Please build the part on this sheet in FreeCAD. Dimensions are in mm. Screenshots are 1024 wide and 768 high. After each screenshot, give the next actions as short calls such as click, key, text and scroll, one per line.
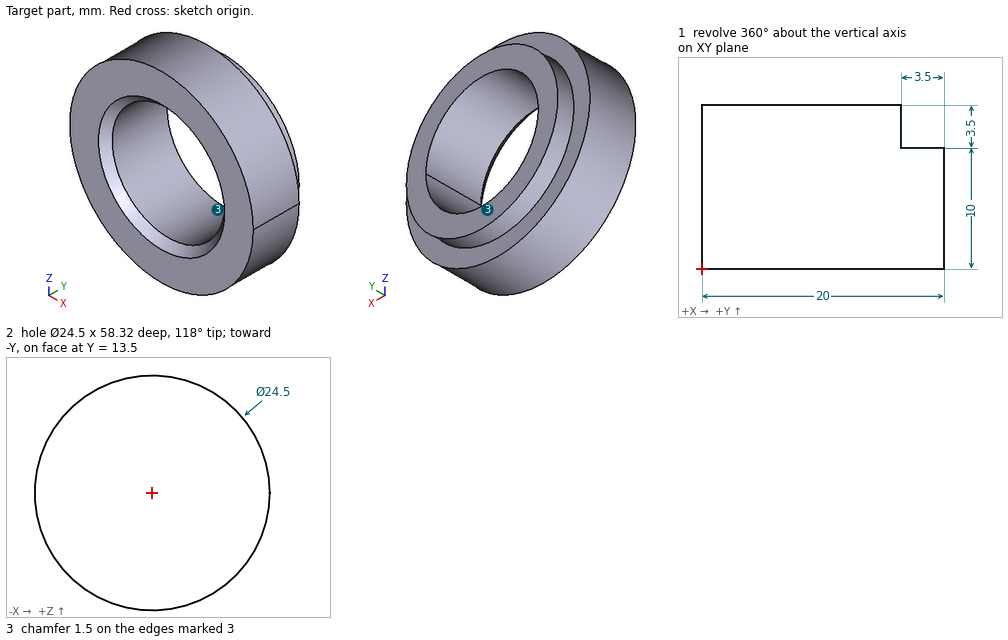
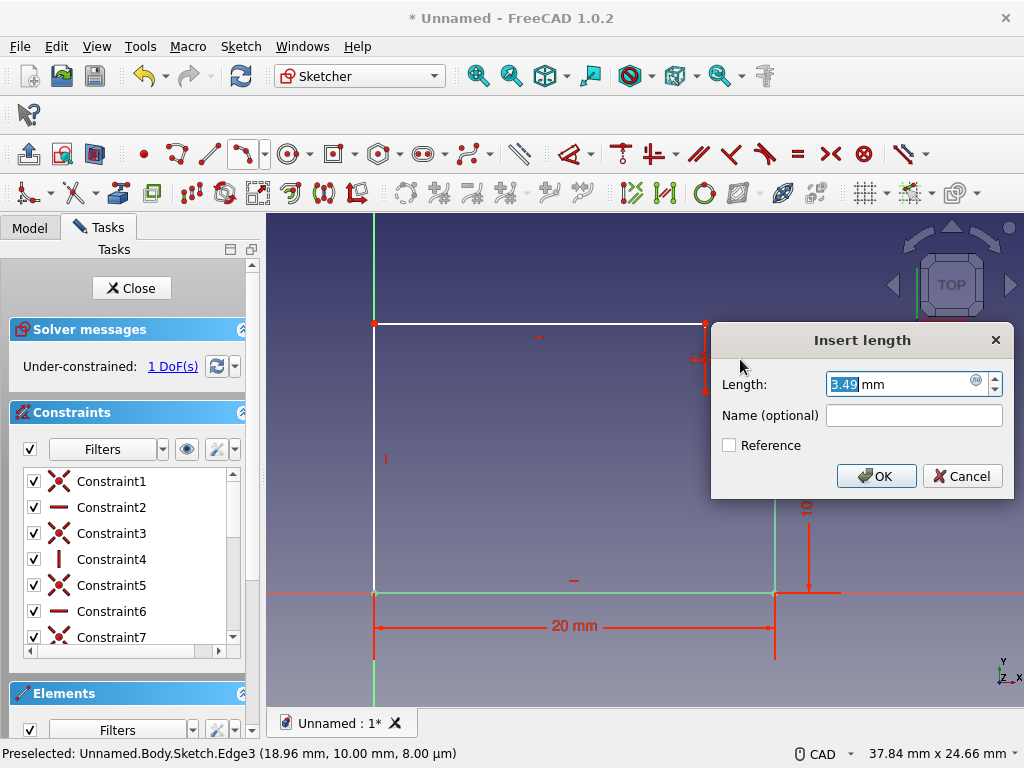
text(3.5)
key(Return)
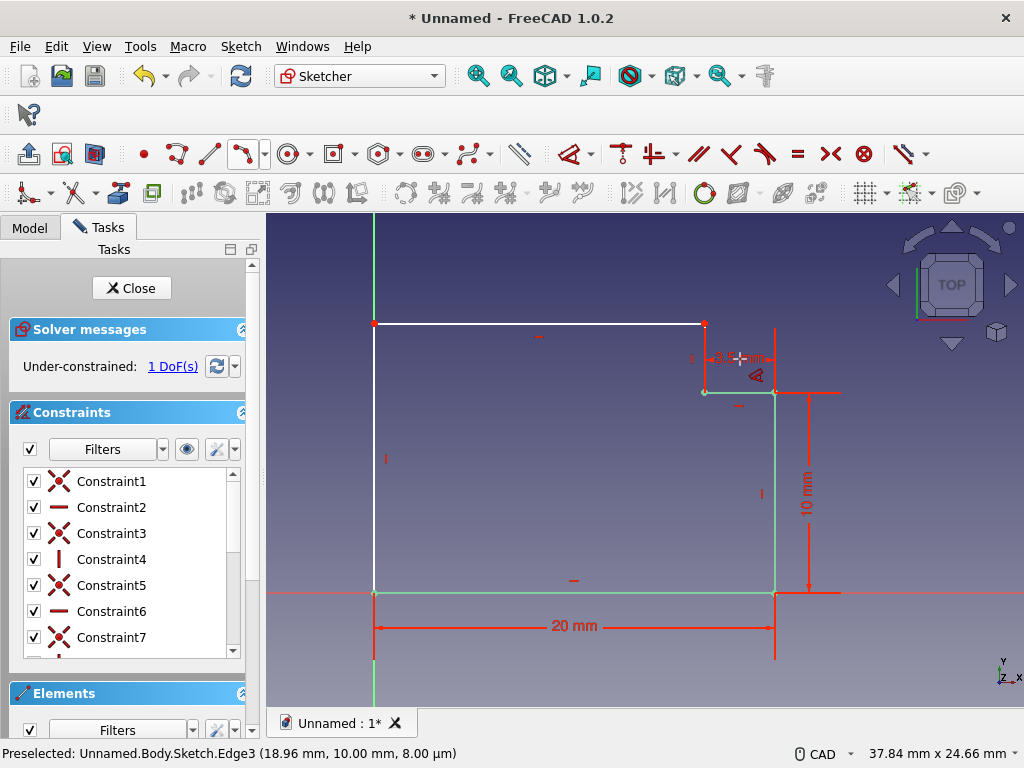
click(705, 372)
click(739, 334)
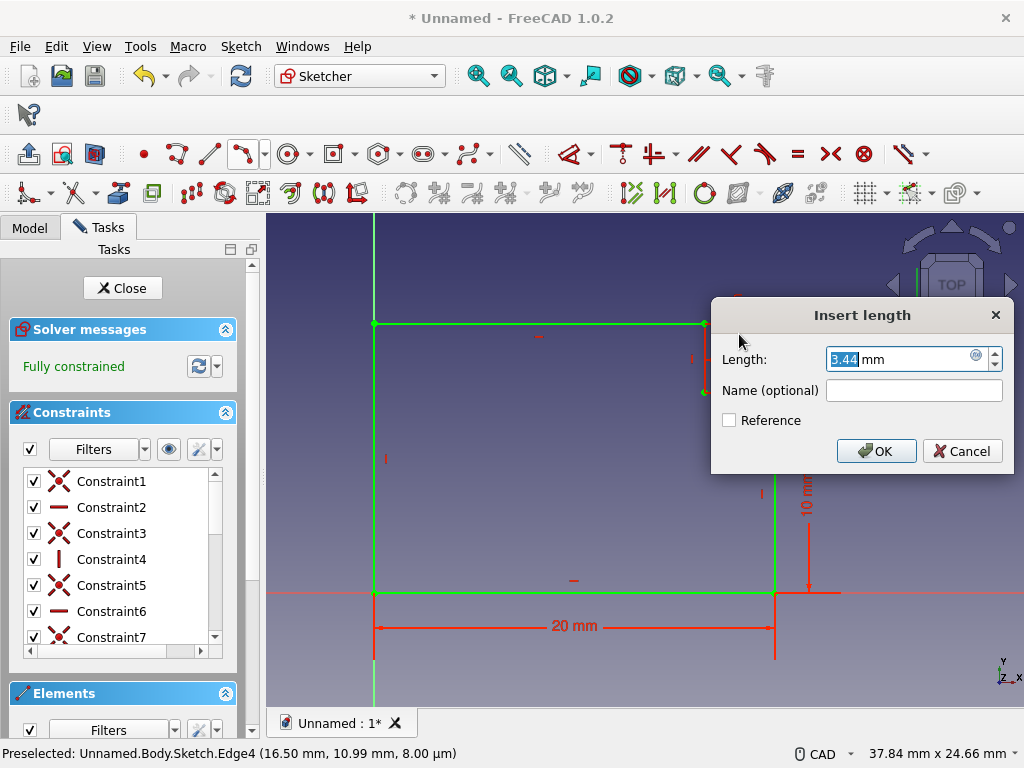
text(3.5)
key(Return)
key(Escape)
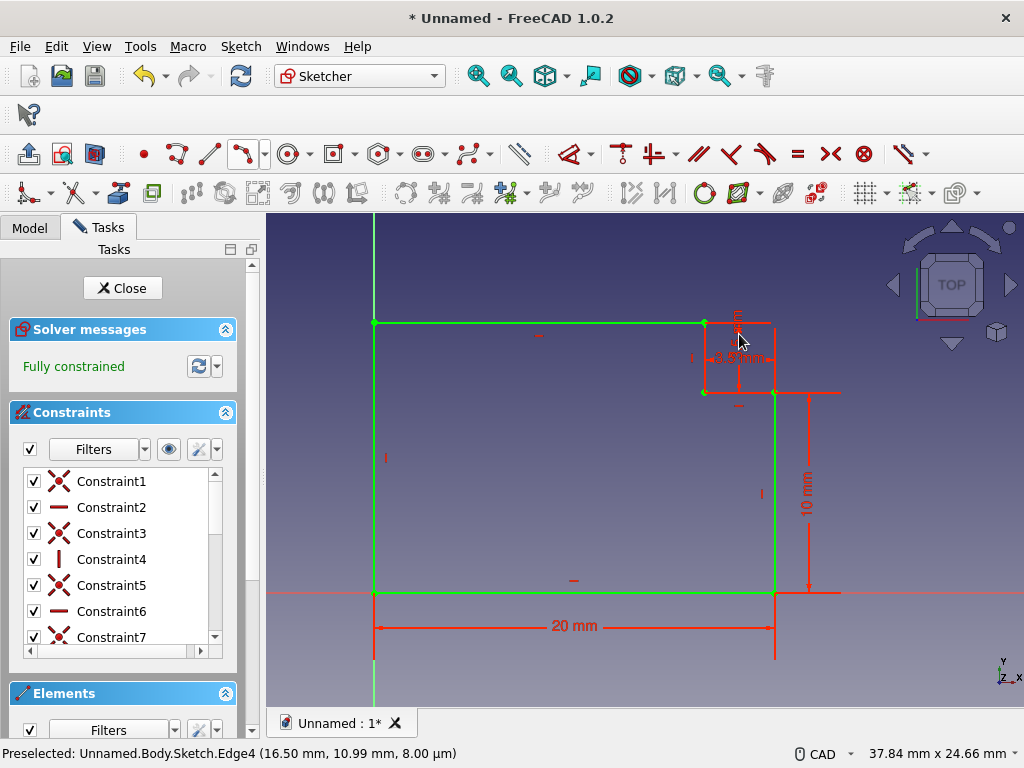
click(123, 288)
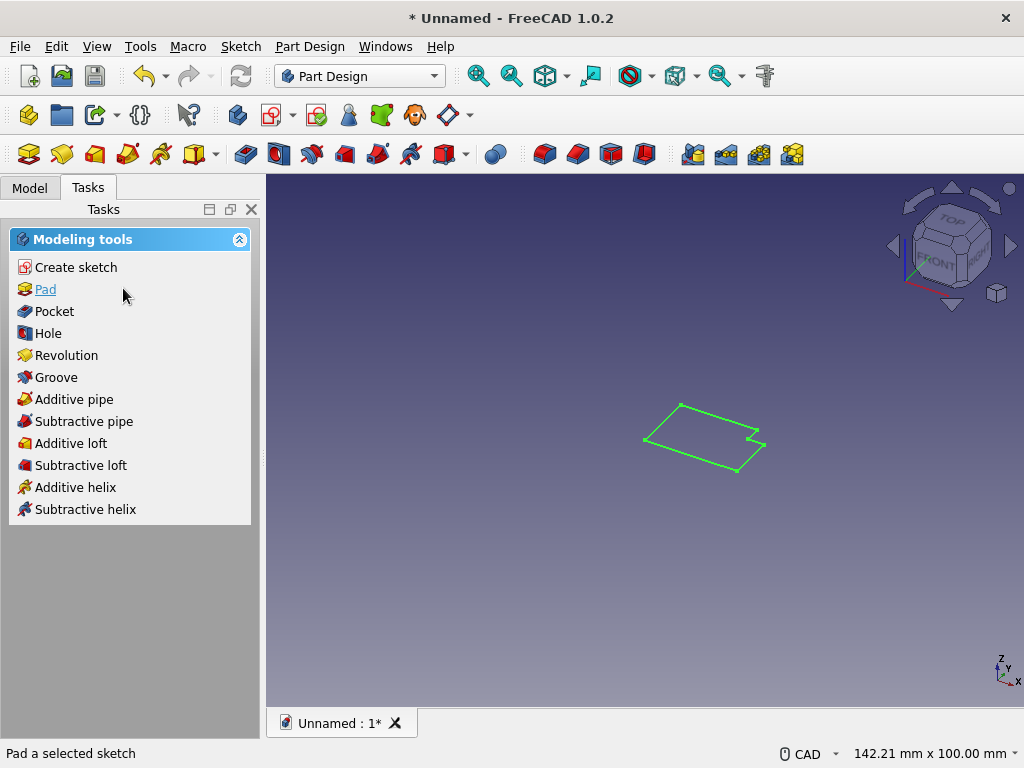
click(62, 154)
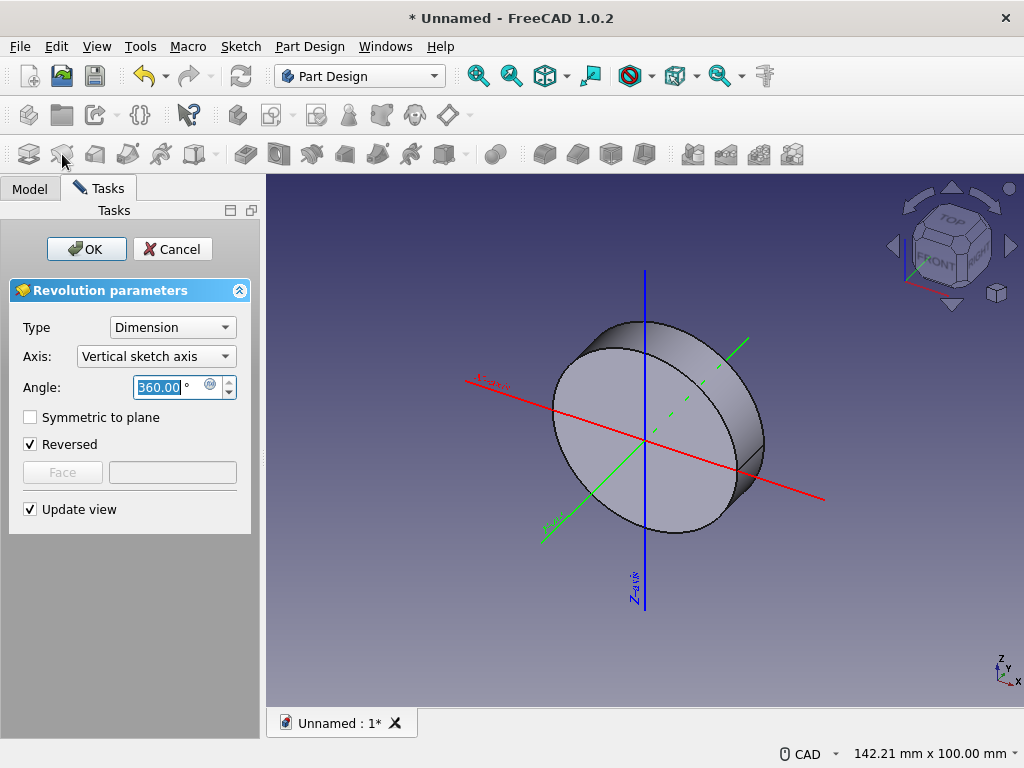
click(87, 249)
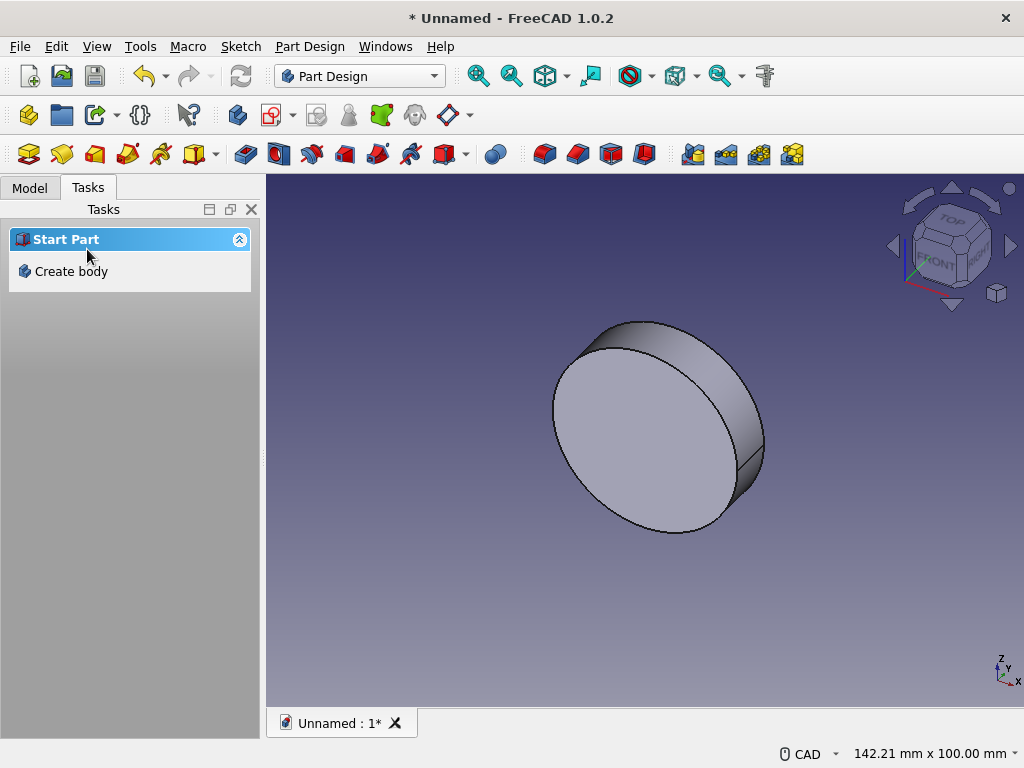
key(4)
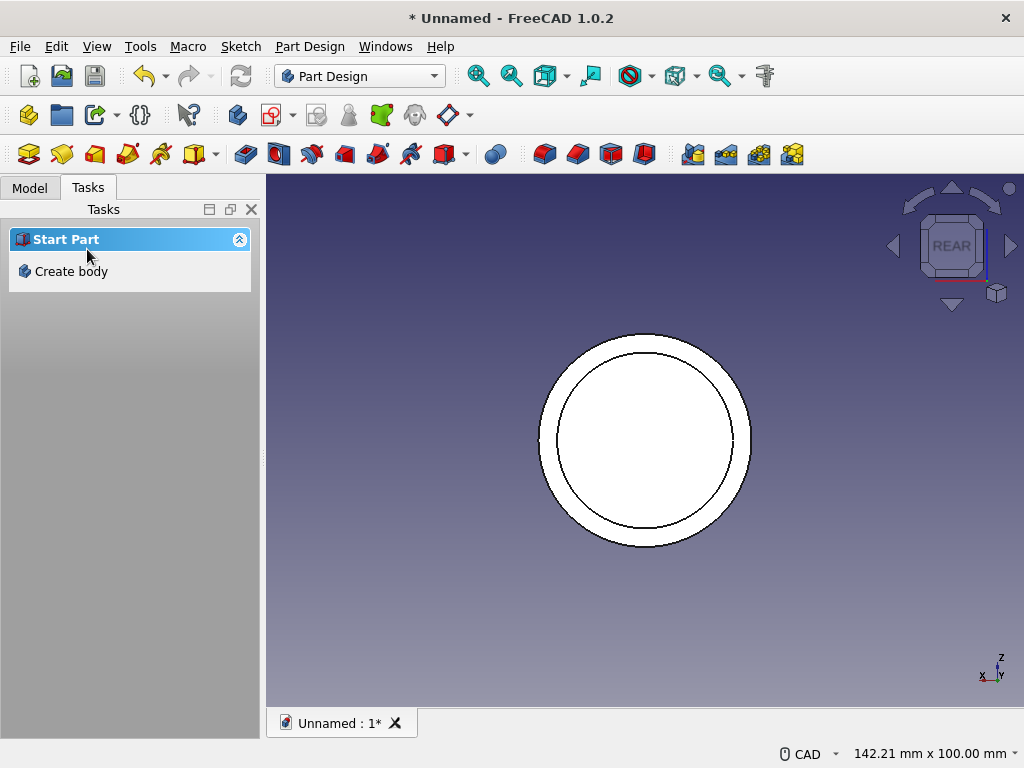
click(479, 76)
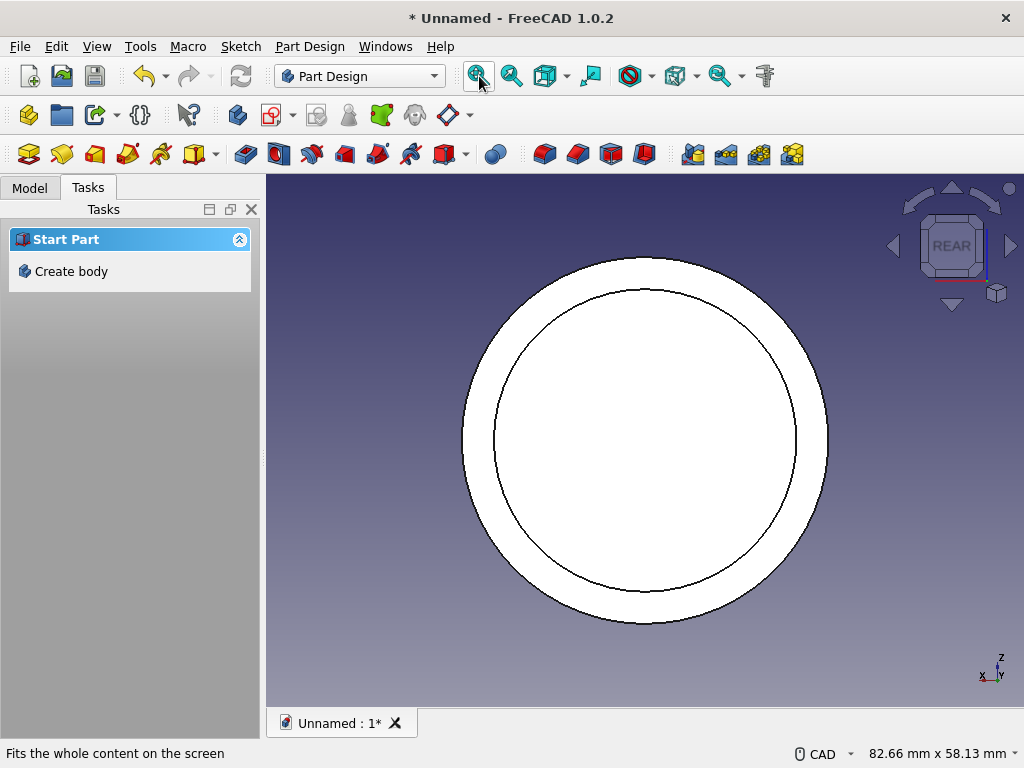
click(645, 440)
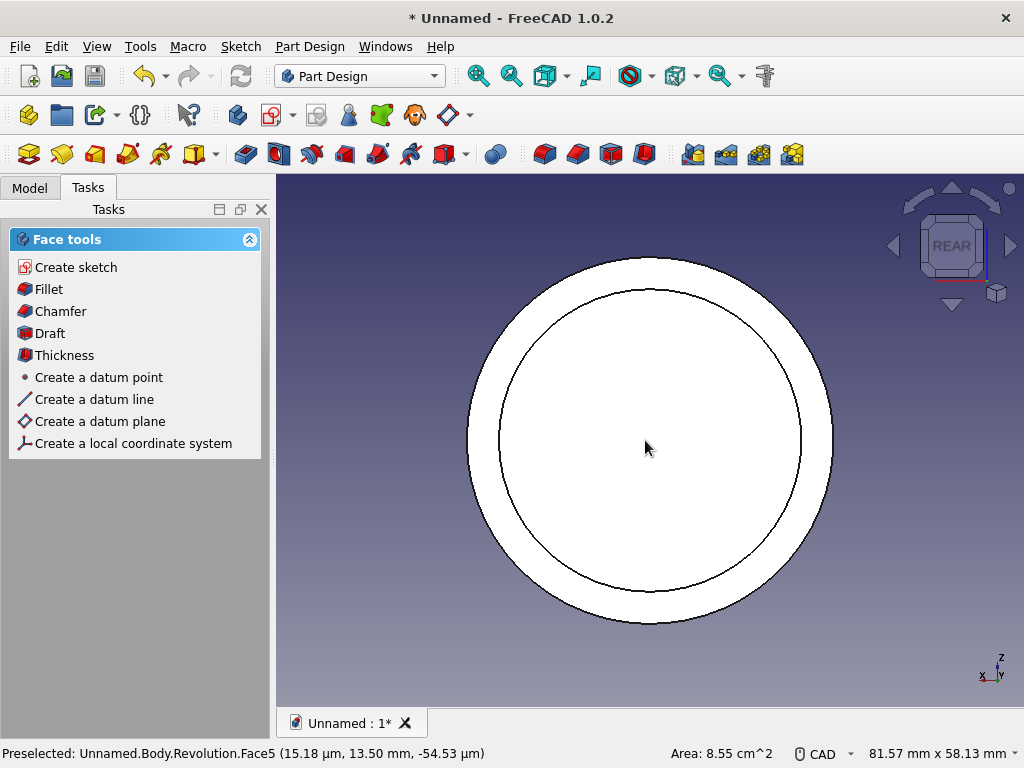
click(270, 116)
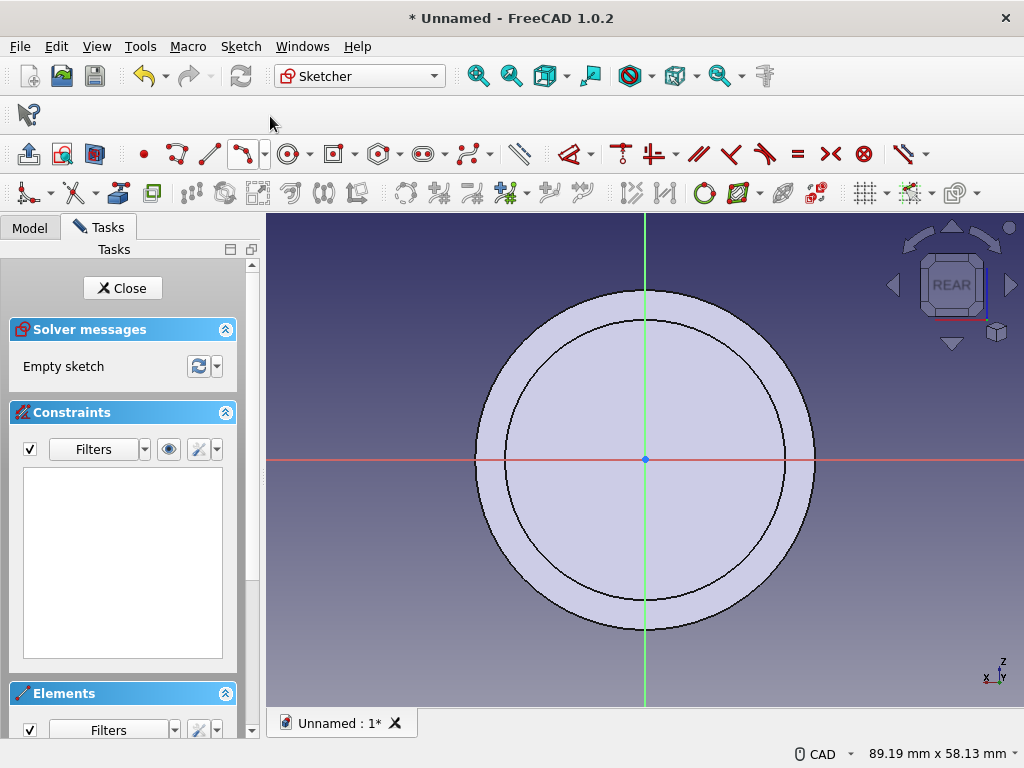
scroll(785, 460, up, 2)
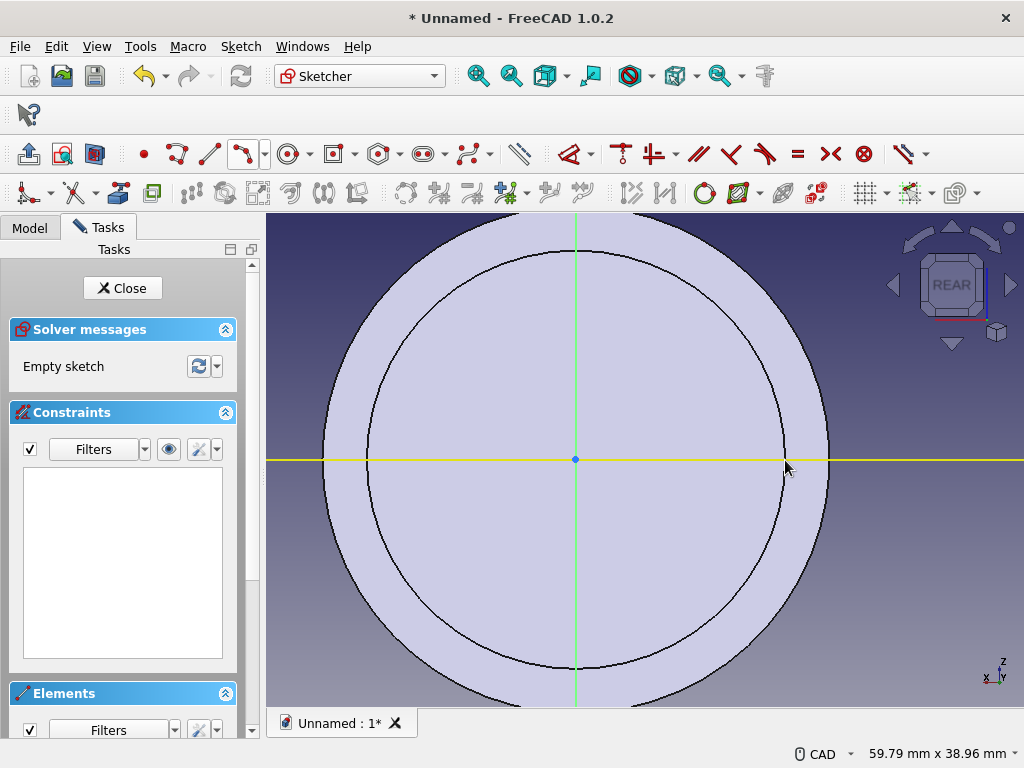
click(288, 154)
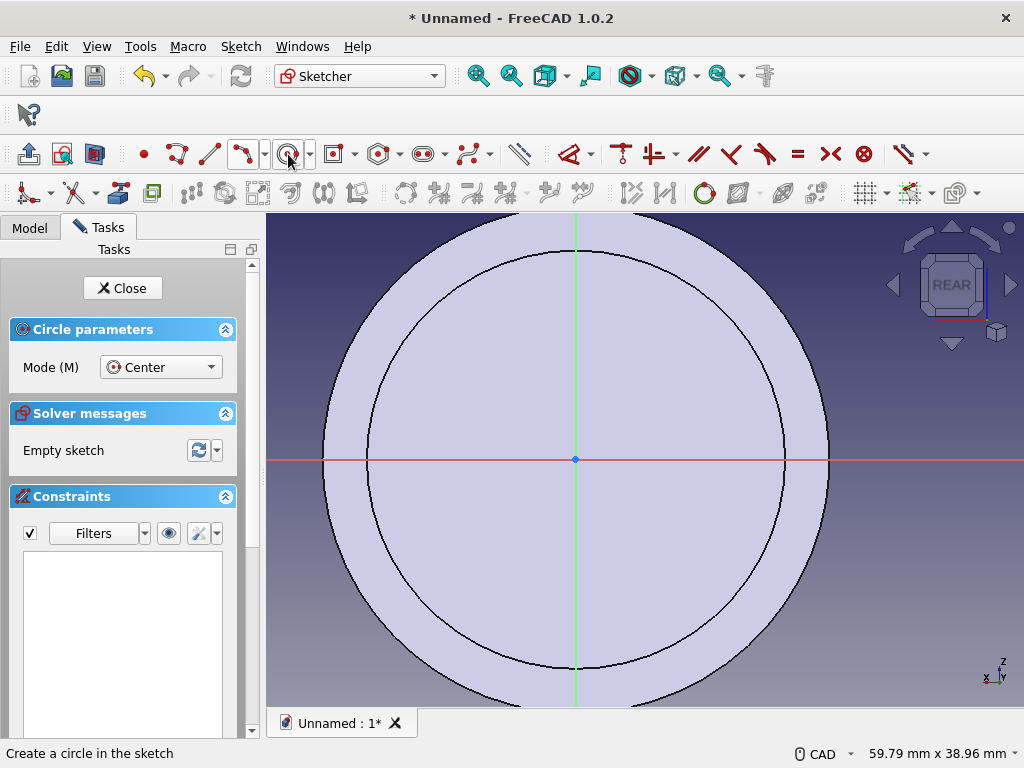
click(576, 460)
move(686, 350)